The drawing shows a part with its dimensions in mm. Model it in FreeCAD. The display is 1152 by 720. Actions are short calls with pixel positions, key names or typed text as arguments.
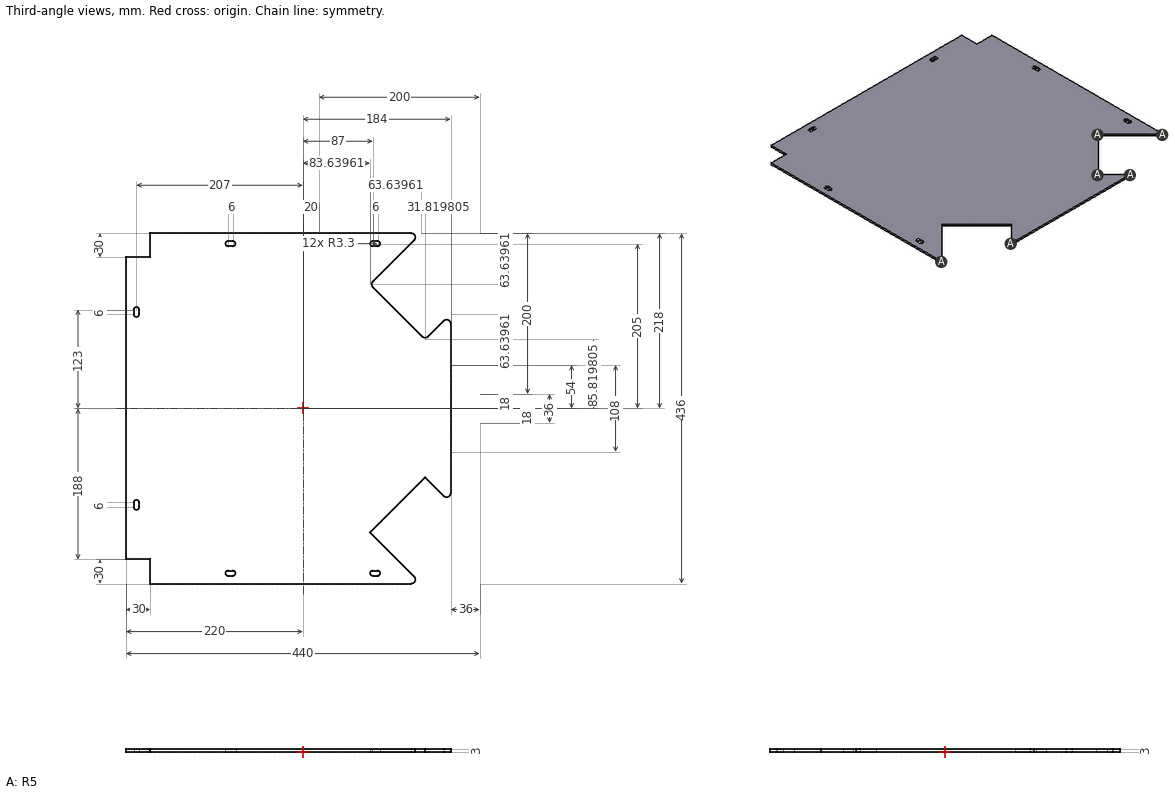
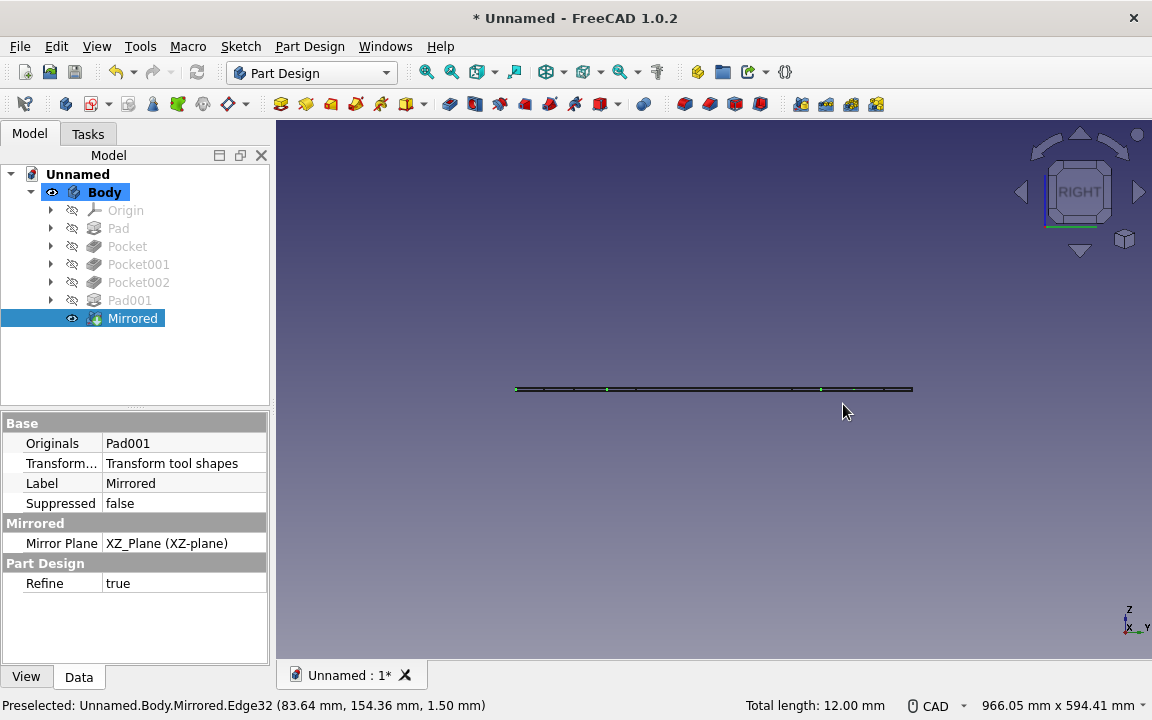
key(5)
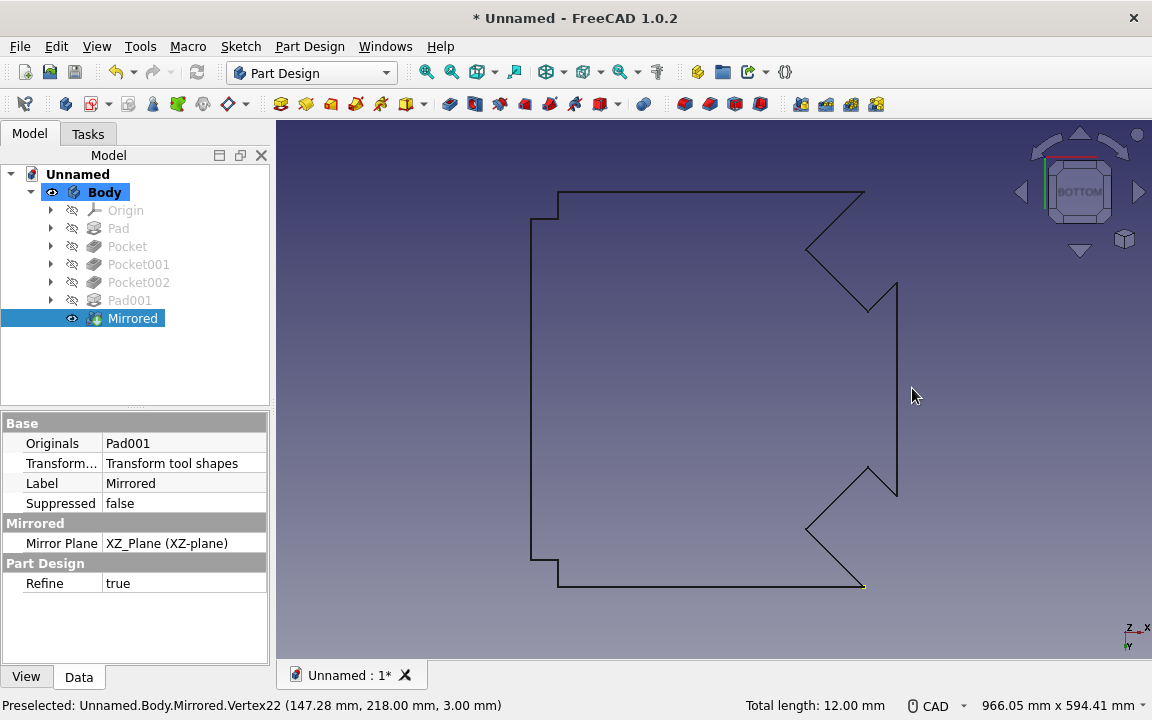
scroll(864, 586, up, 14)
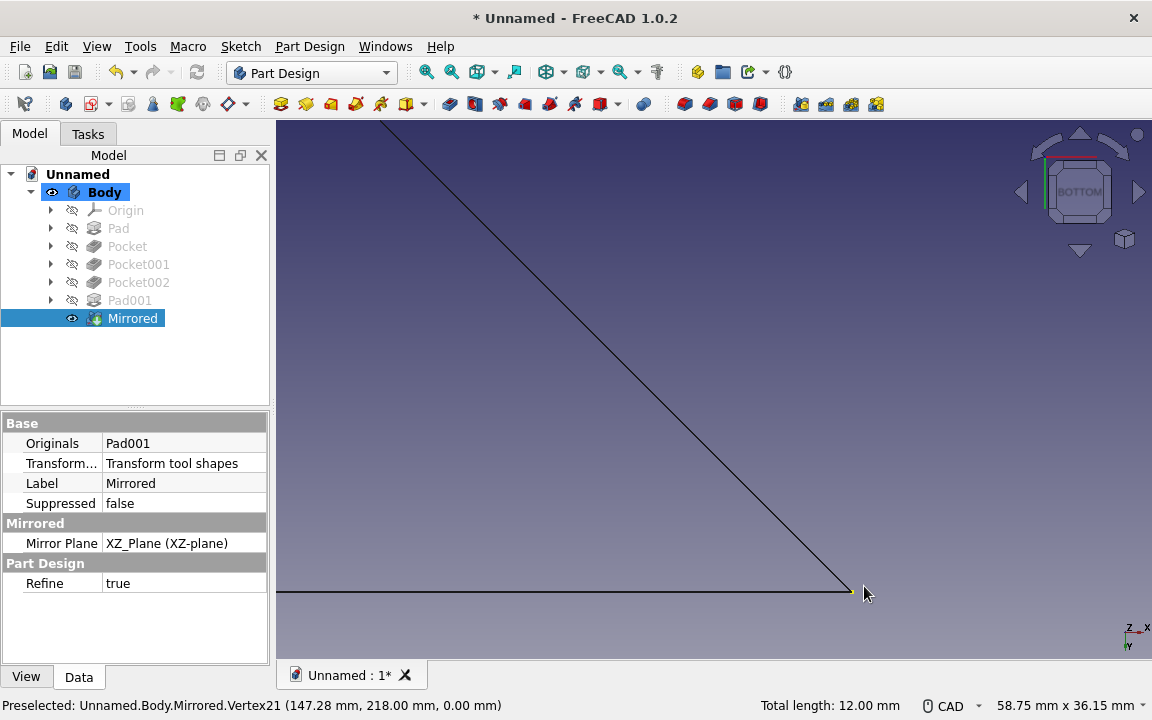
key(v)
key(f)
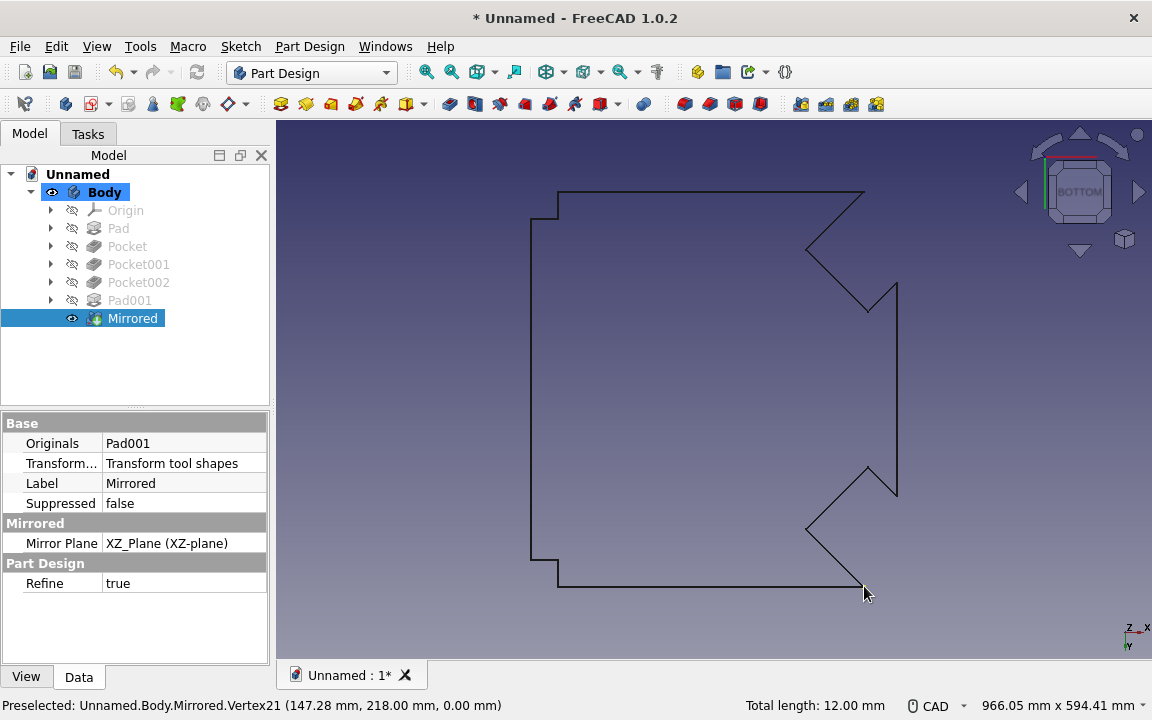
key(4)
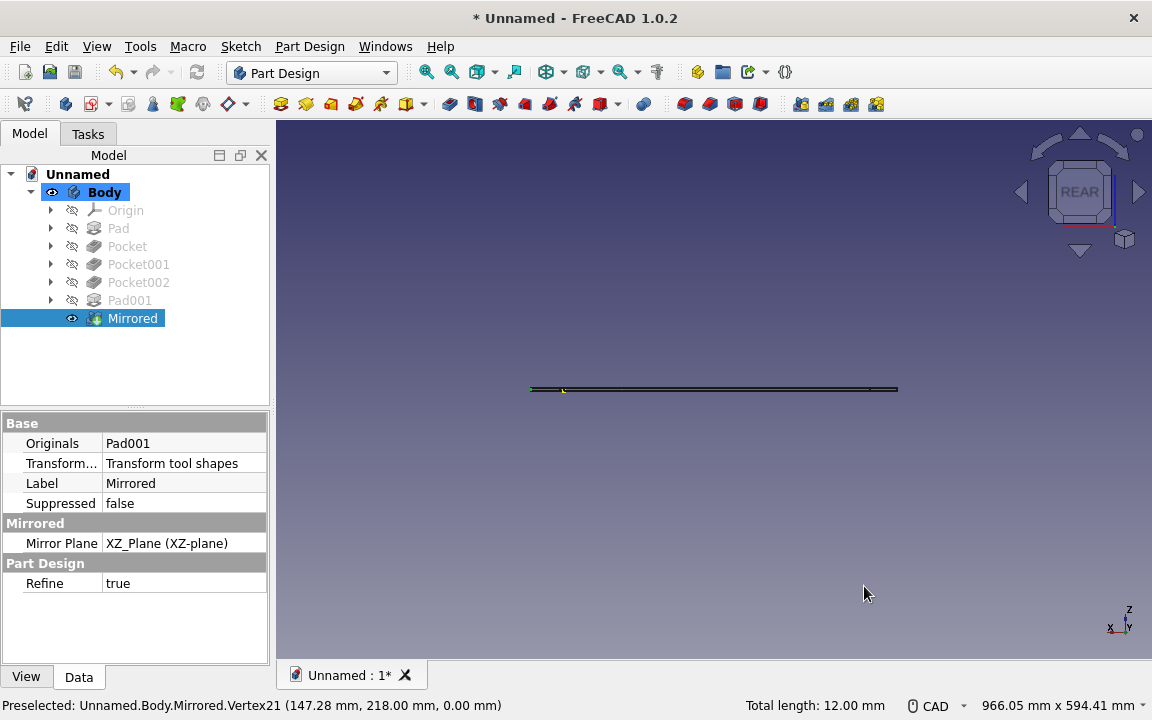
click(427, 72)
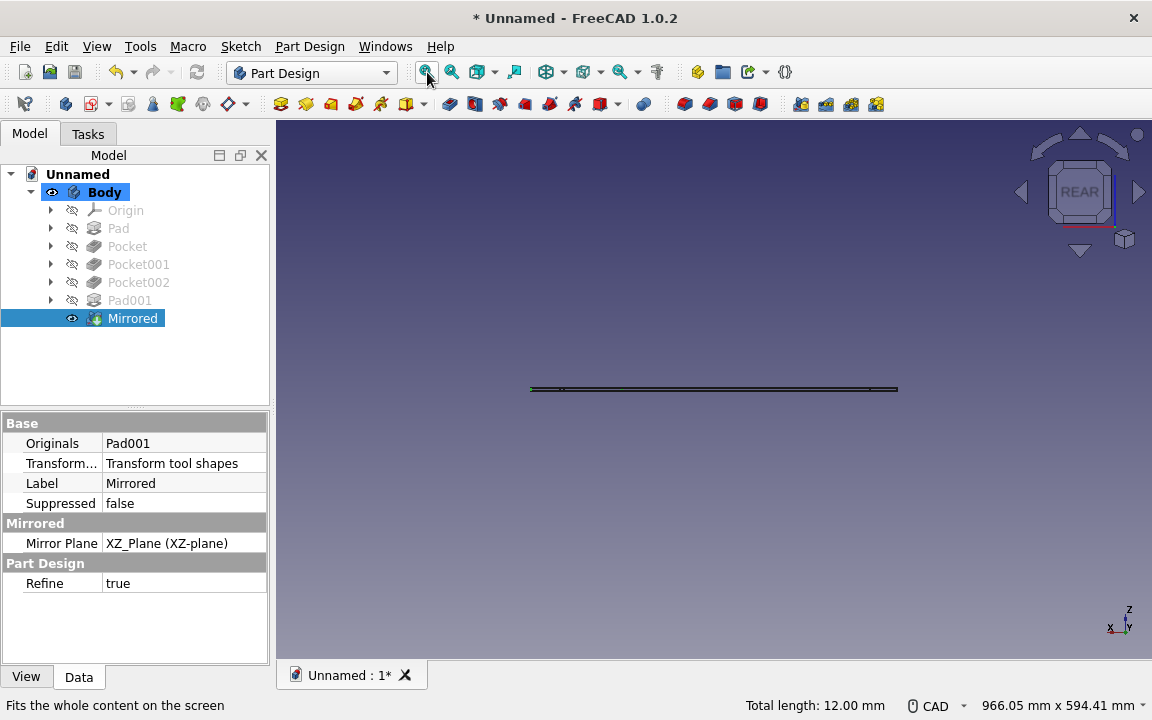
scroll(564, 389, up, 14)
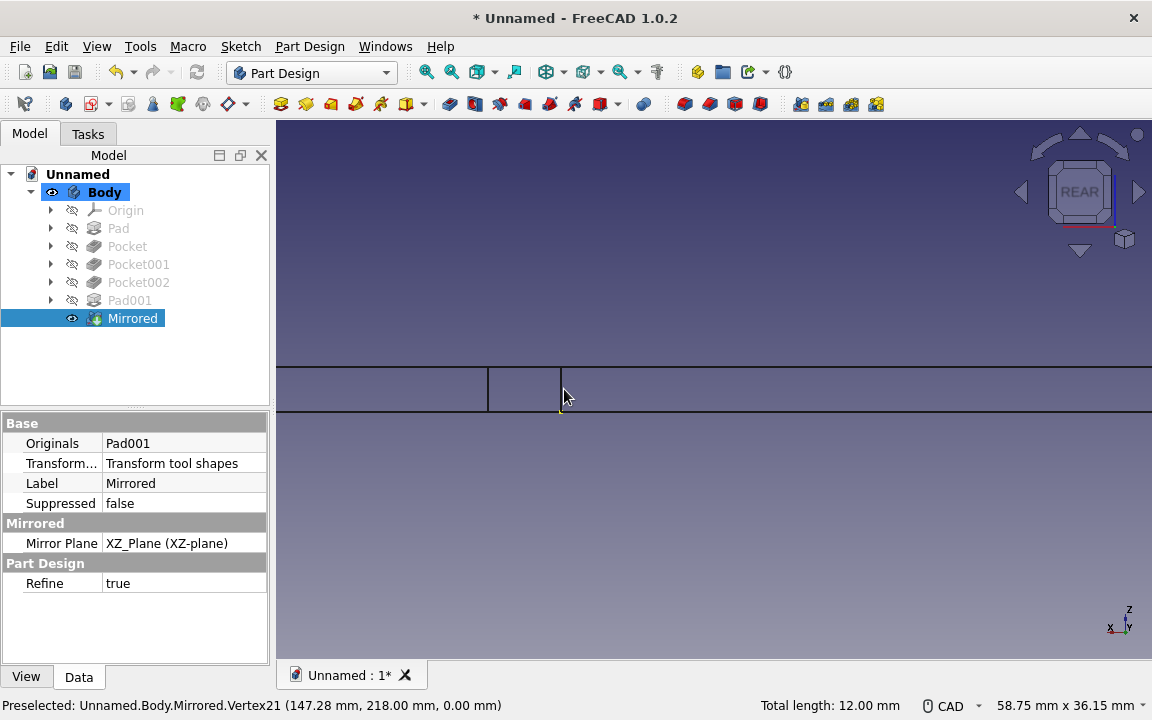
click(561, 389, ctrl)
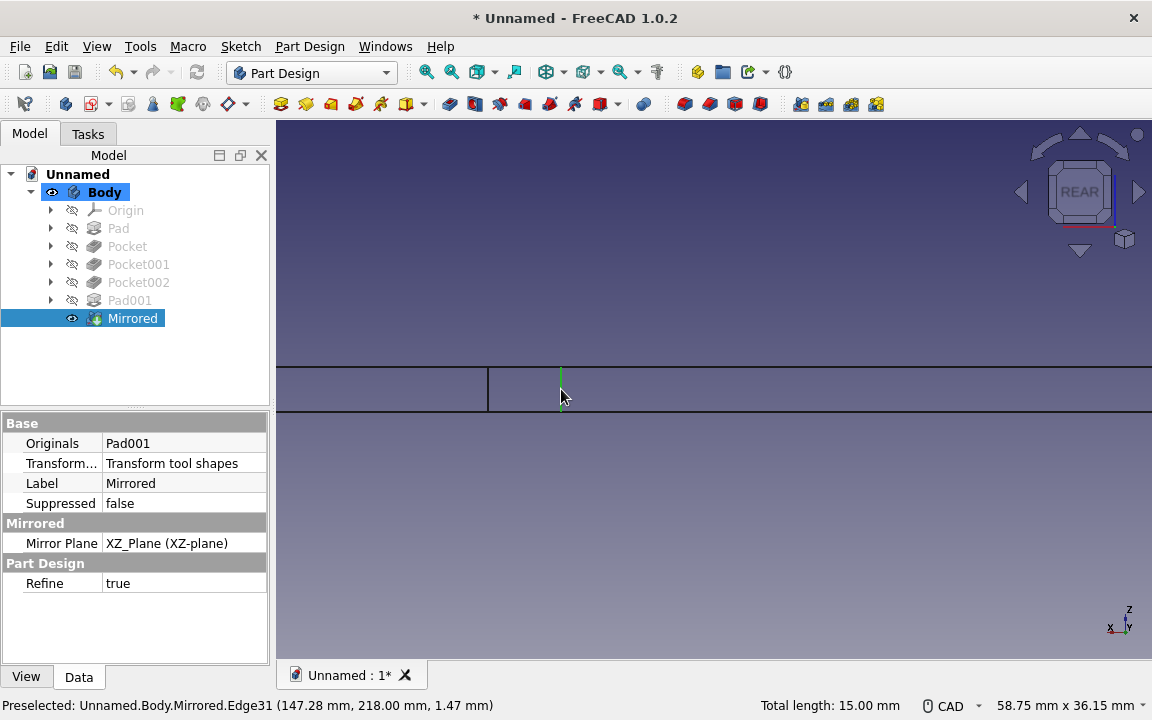
click(488, 389, ctrl)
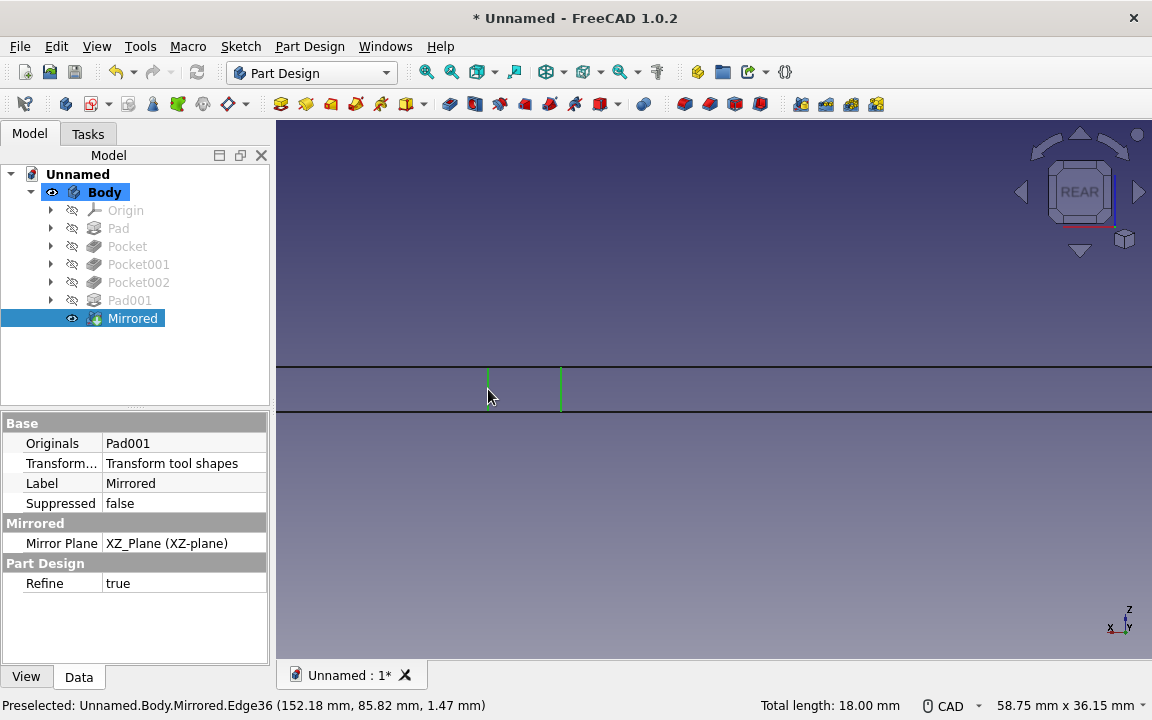
key(v)
key(1)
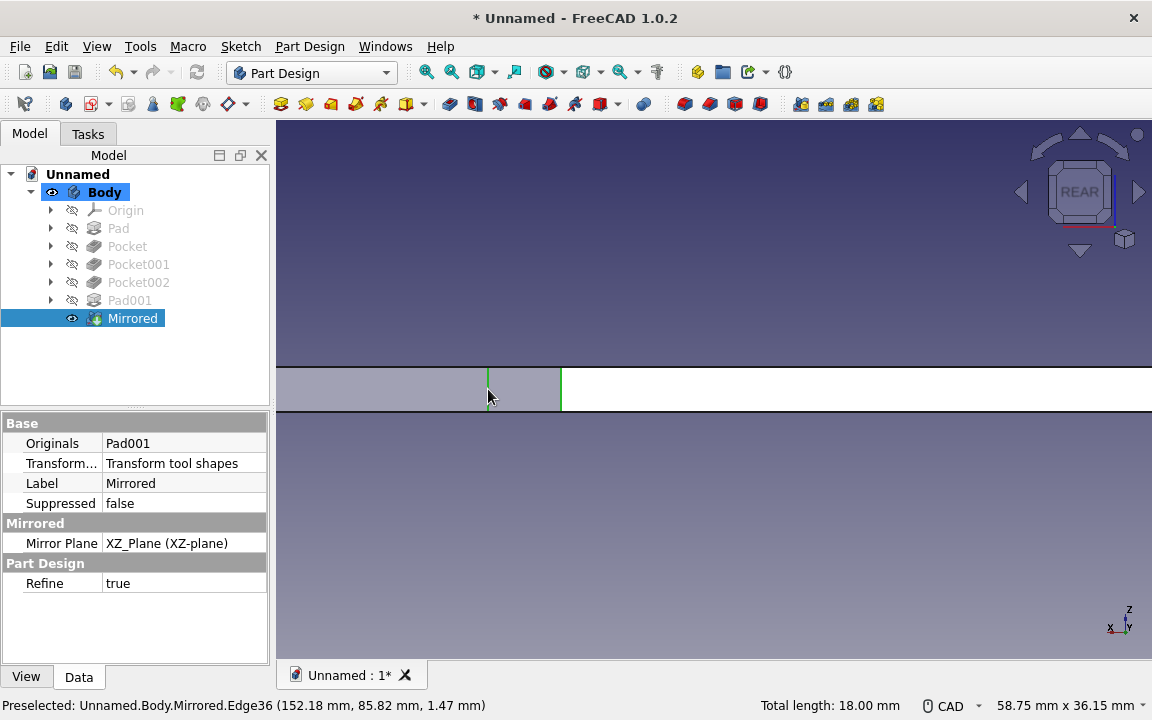
click(685, 104)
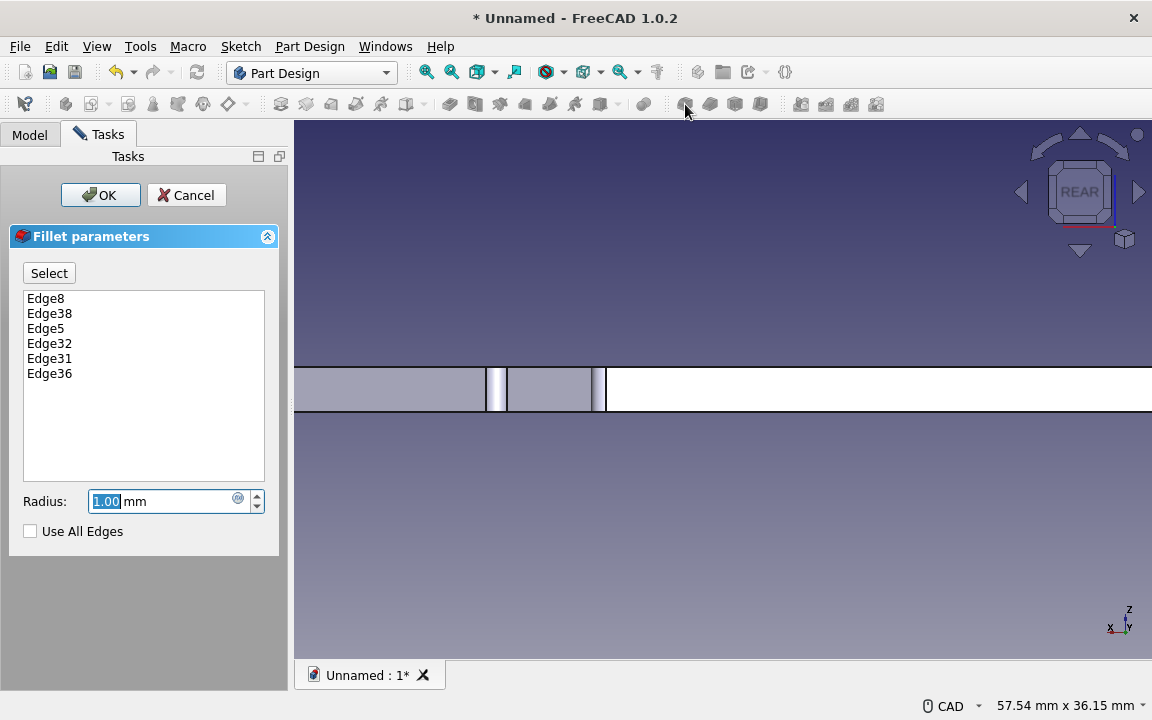
text(5)
key(Tab)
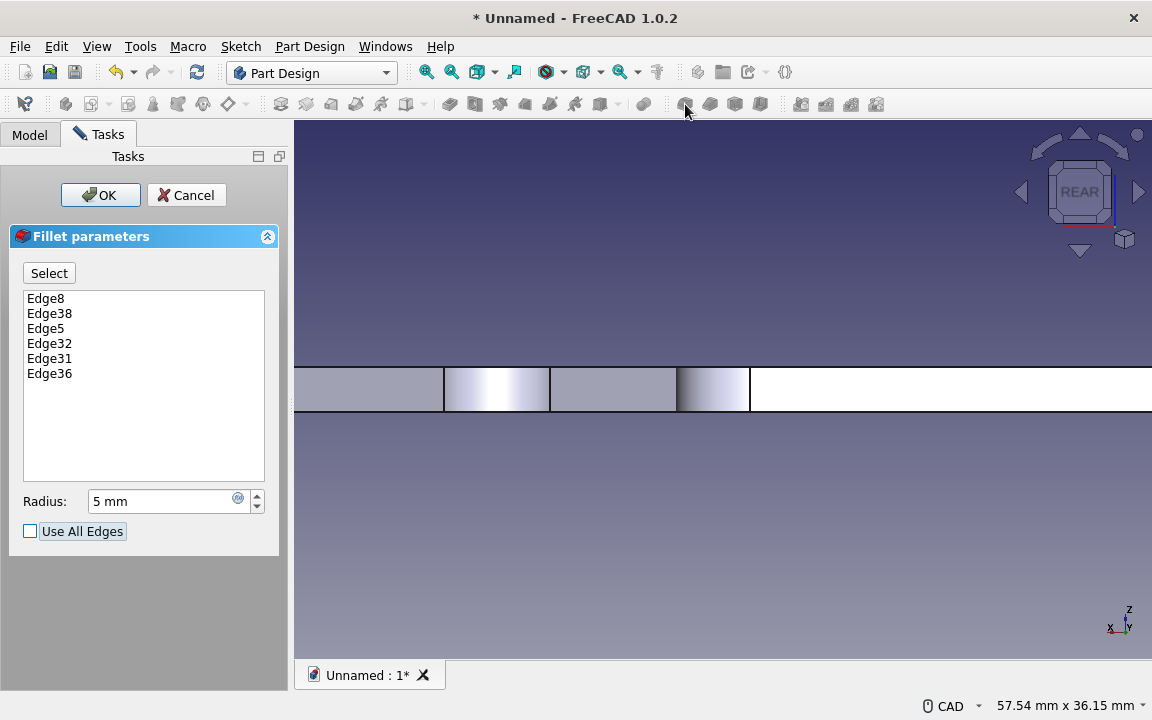
click(101, 195)